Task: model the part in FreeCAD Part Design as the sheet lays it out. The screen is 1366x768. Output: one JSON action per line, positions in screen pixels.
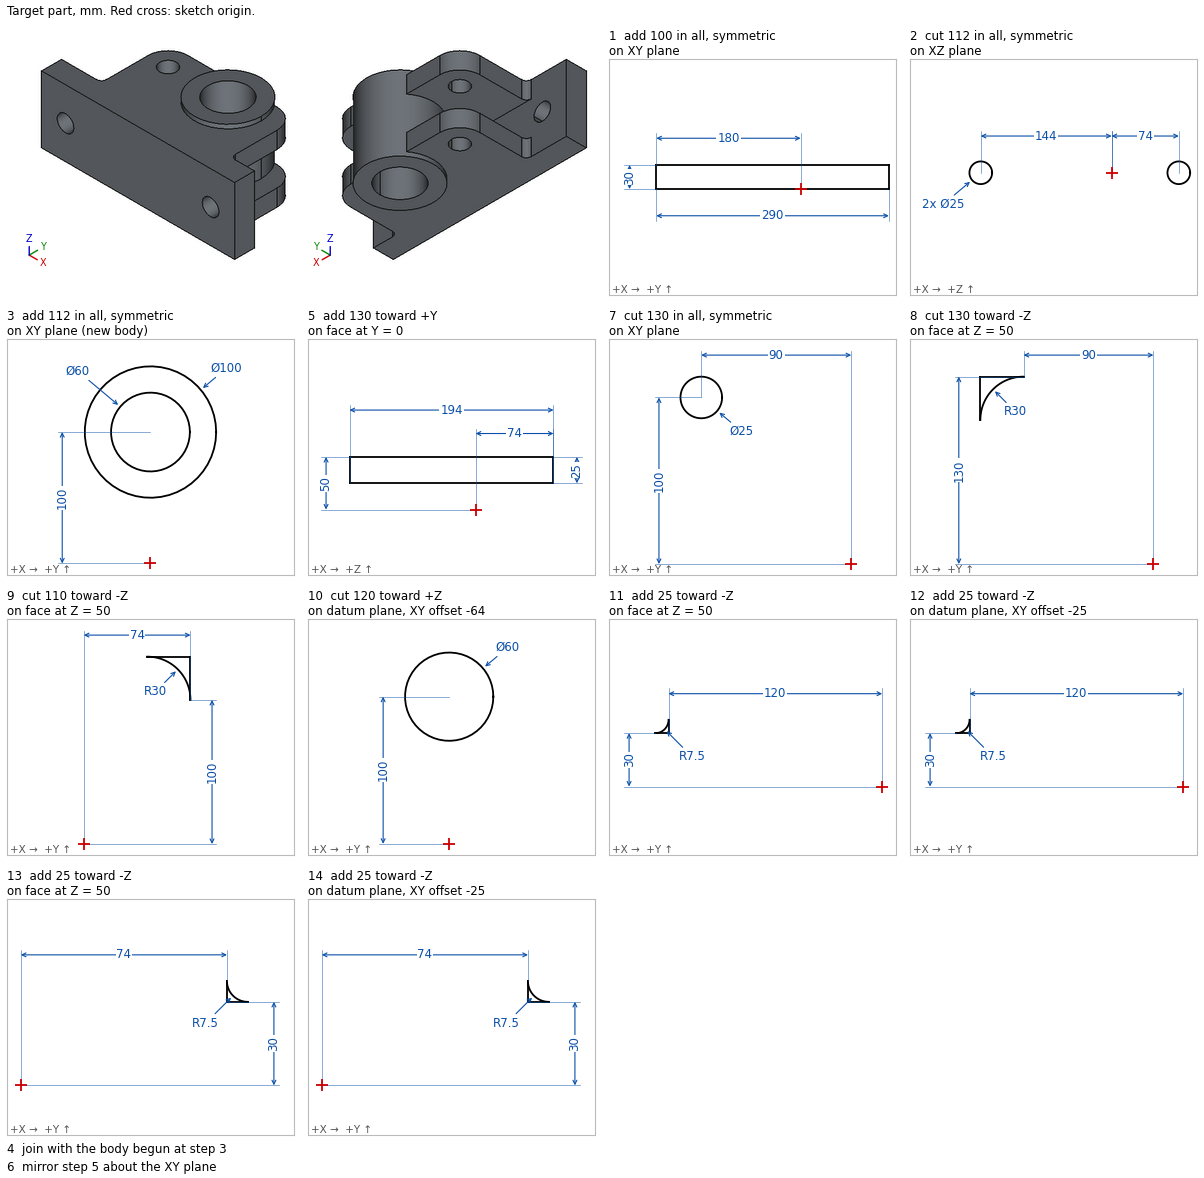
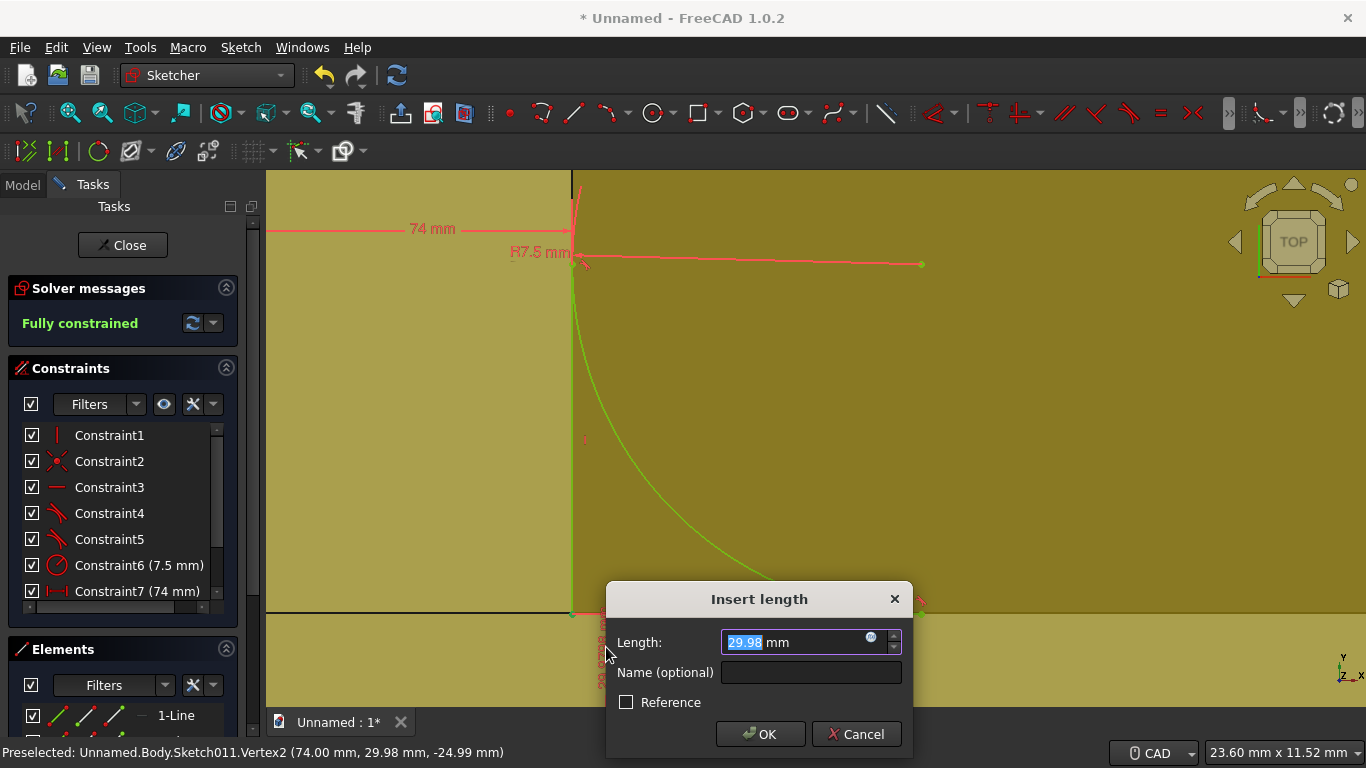
{"action": "type", "text": "30"}
{"action": "key", "text": "Return"}
{"action": "key", "text": "Escape"}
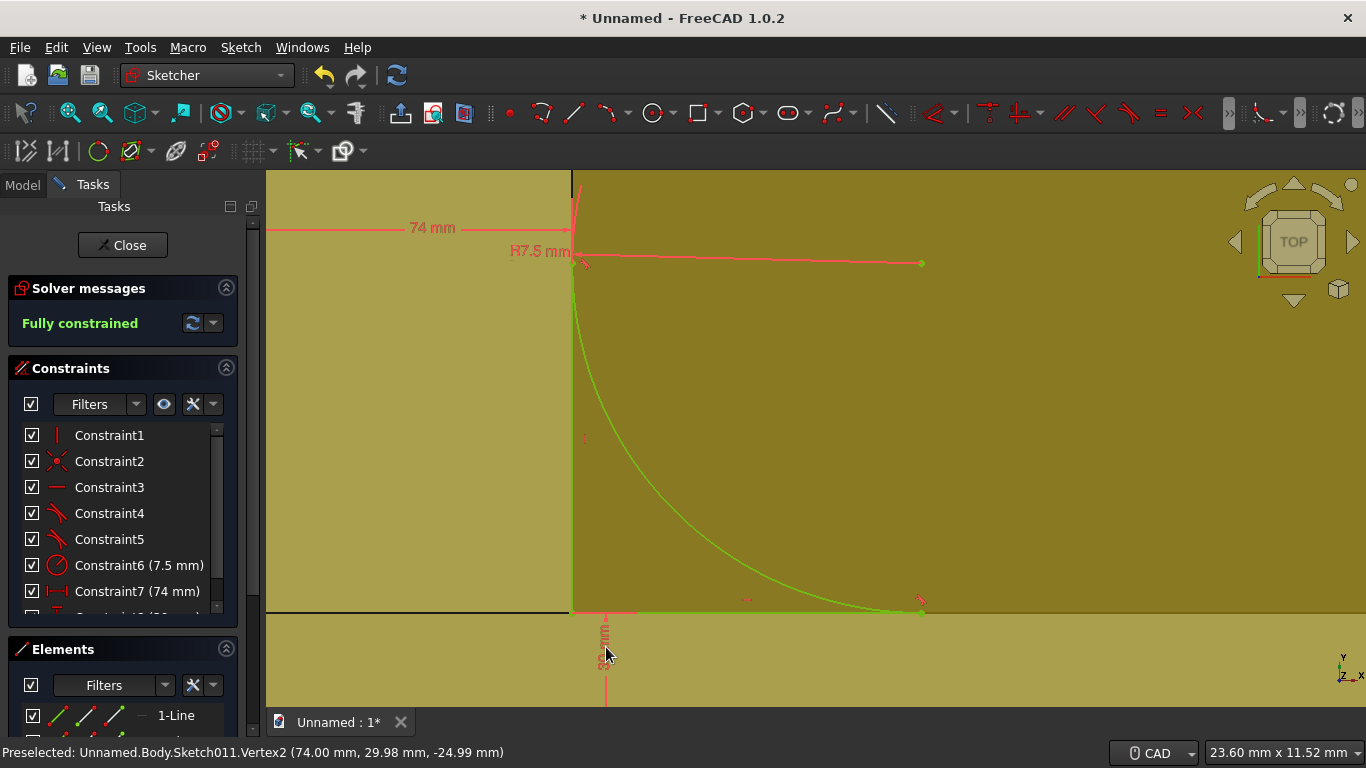
{"action": "left_click", "coordinate": [123, 245]}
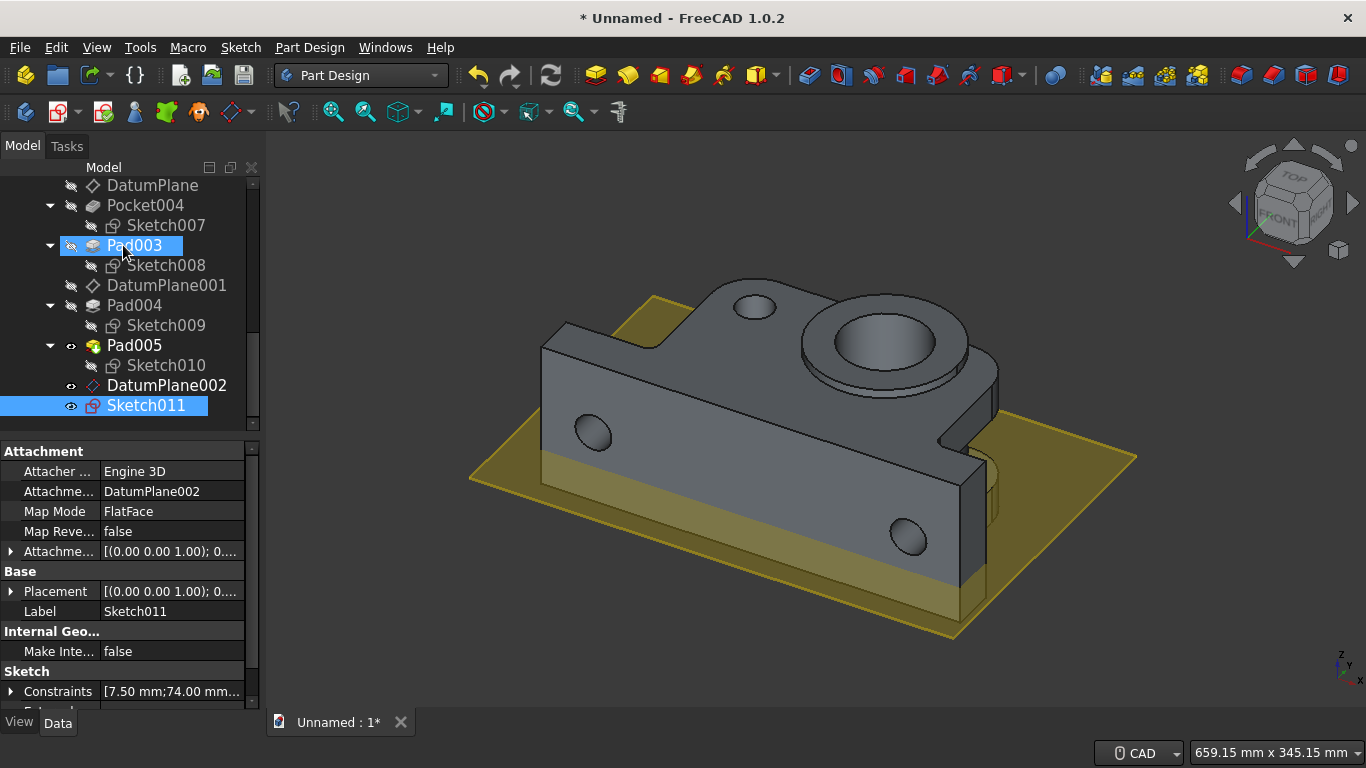
{"action": "left_click", "coordinate": [596, 76]}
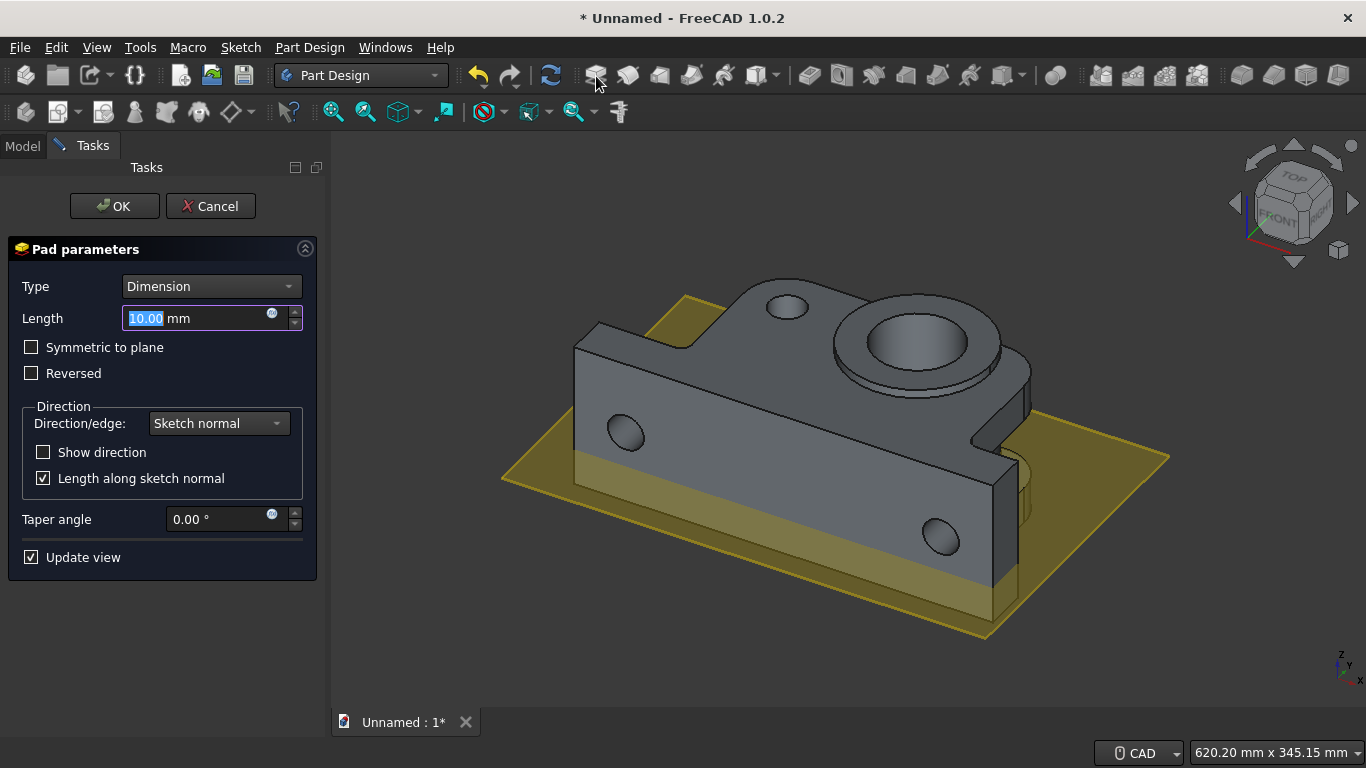
{"action": "type", "text": "25"}
{"action": "key", "text": "Tab"}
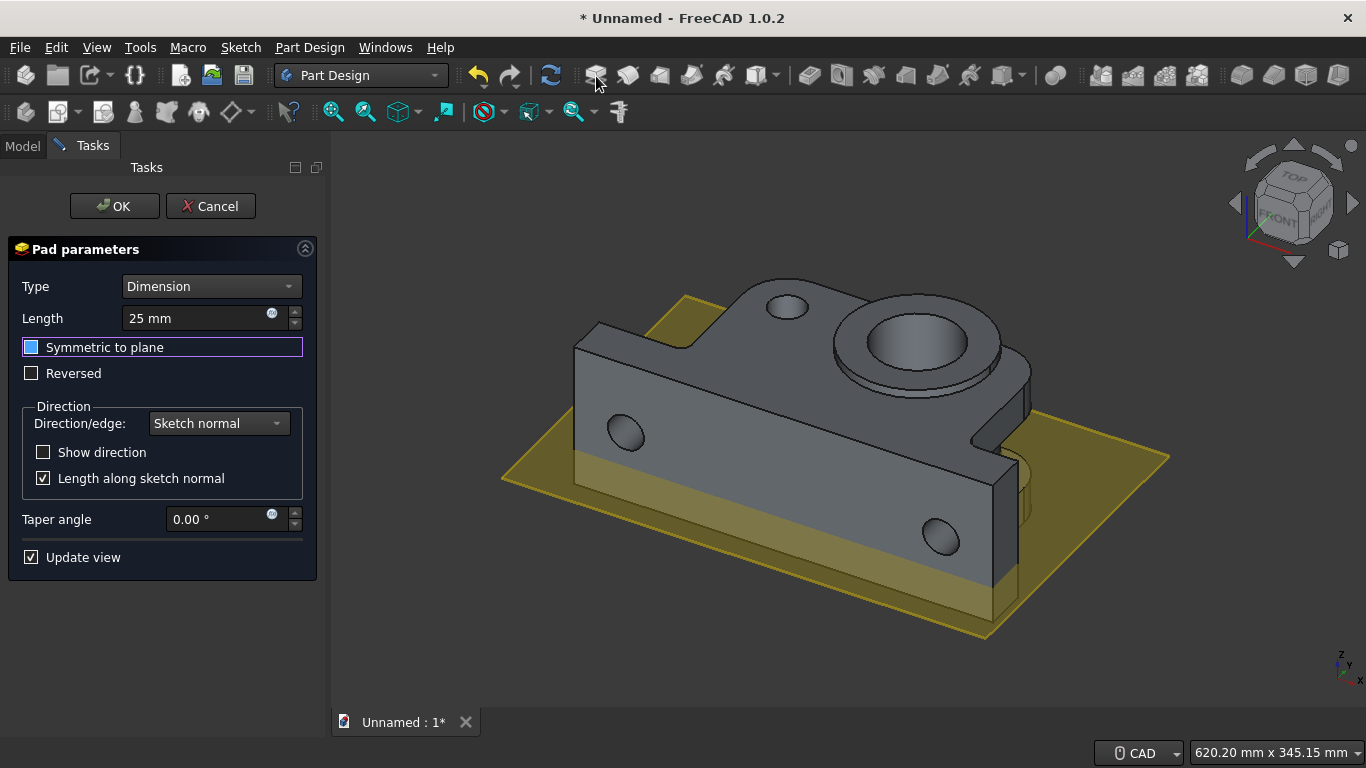
{"action": "left_click", "coordinate": [30, 373]}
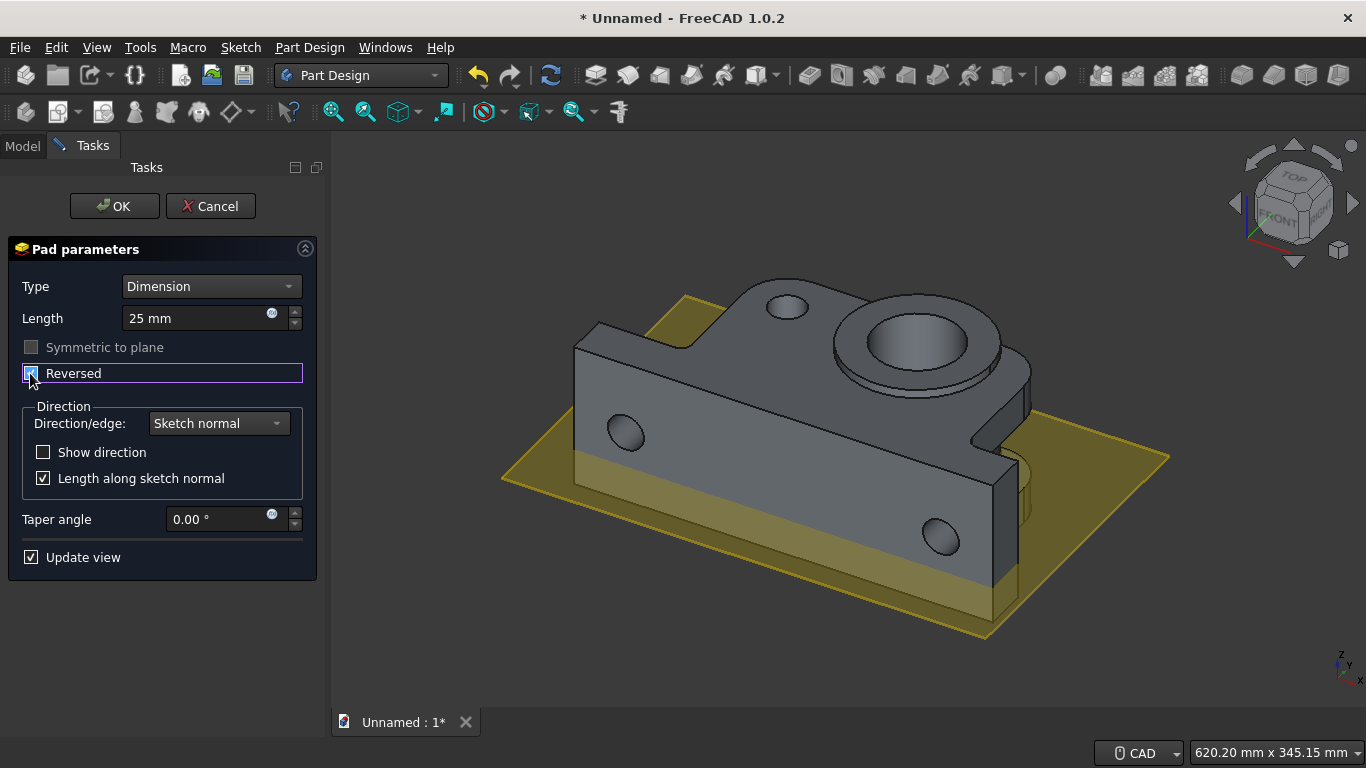
{"action": "left_click", "coordinate": [115, 206]}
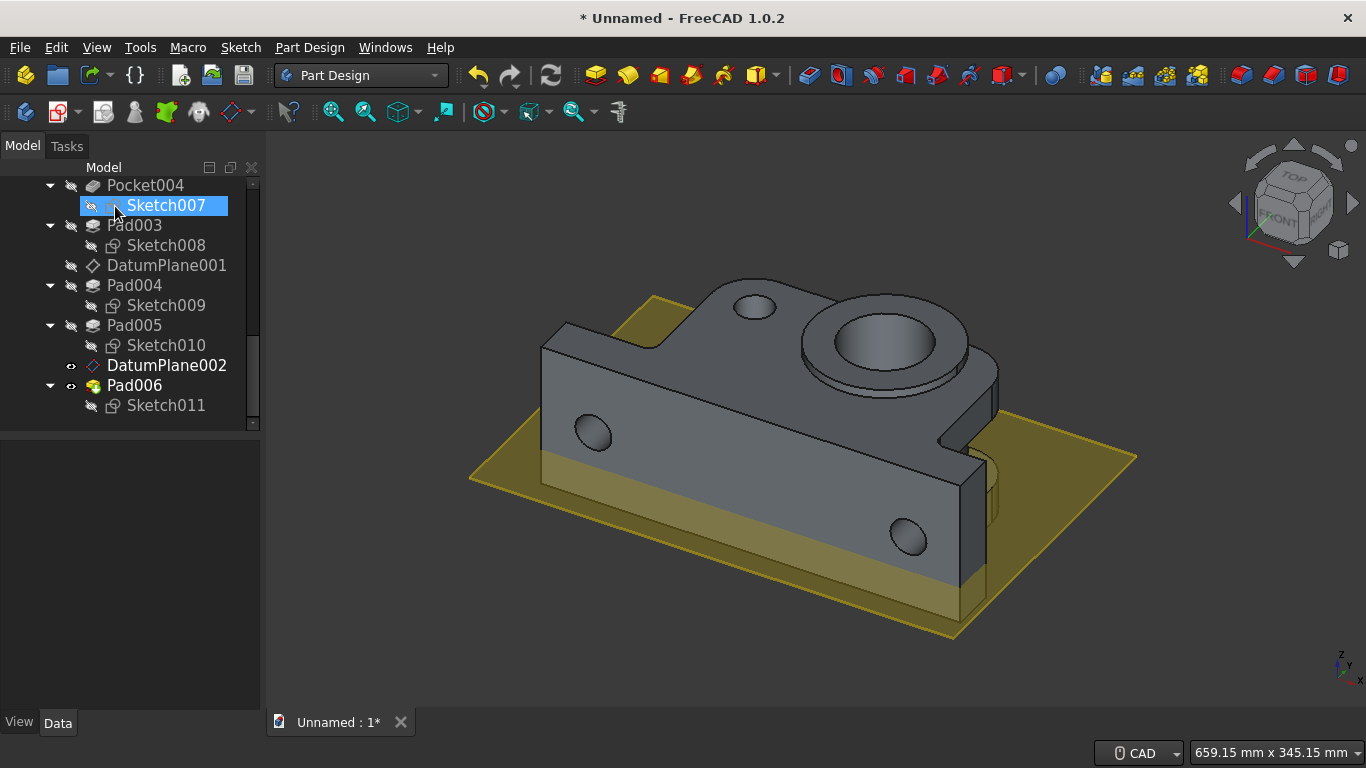
{"action": "left_click", "coordinate": [116, 366]}
{"action": "key", "text": "space"}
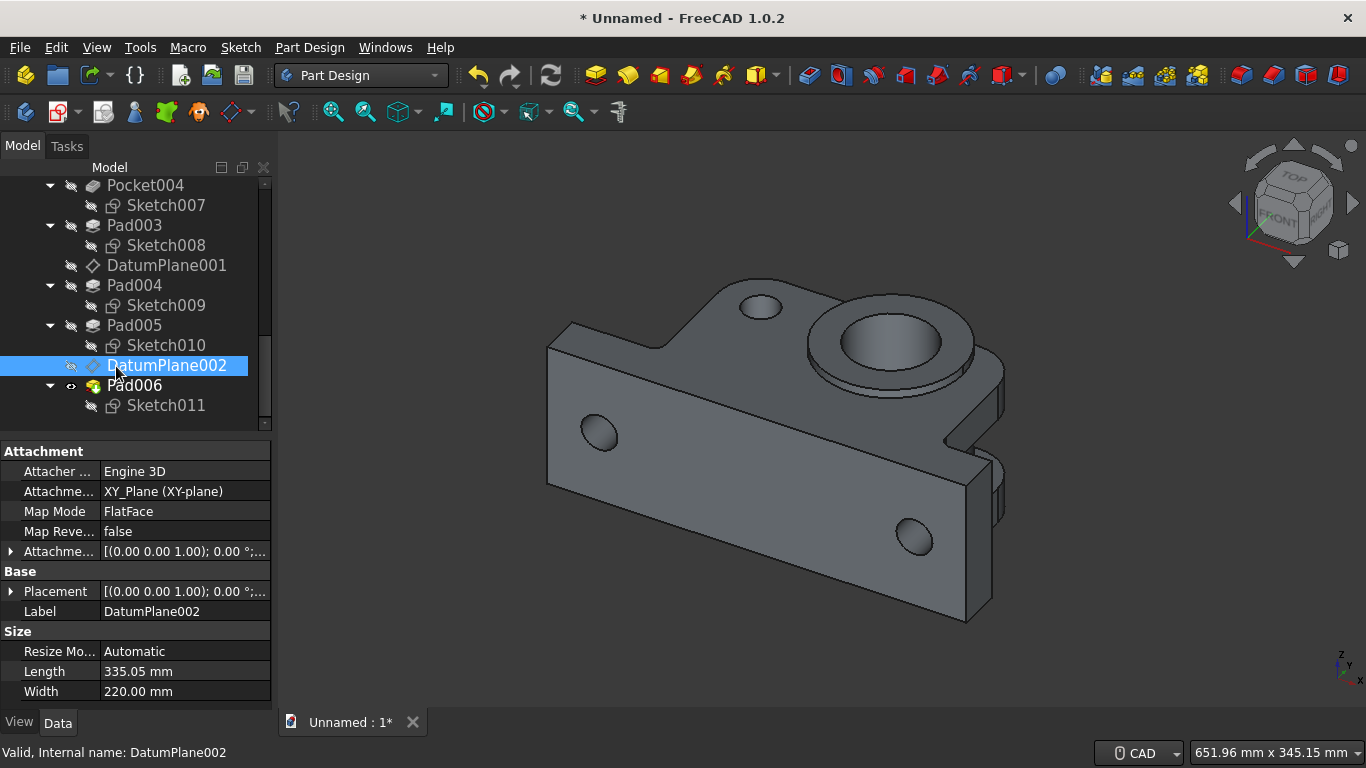
{"action": "key", "text": "0"}